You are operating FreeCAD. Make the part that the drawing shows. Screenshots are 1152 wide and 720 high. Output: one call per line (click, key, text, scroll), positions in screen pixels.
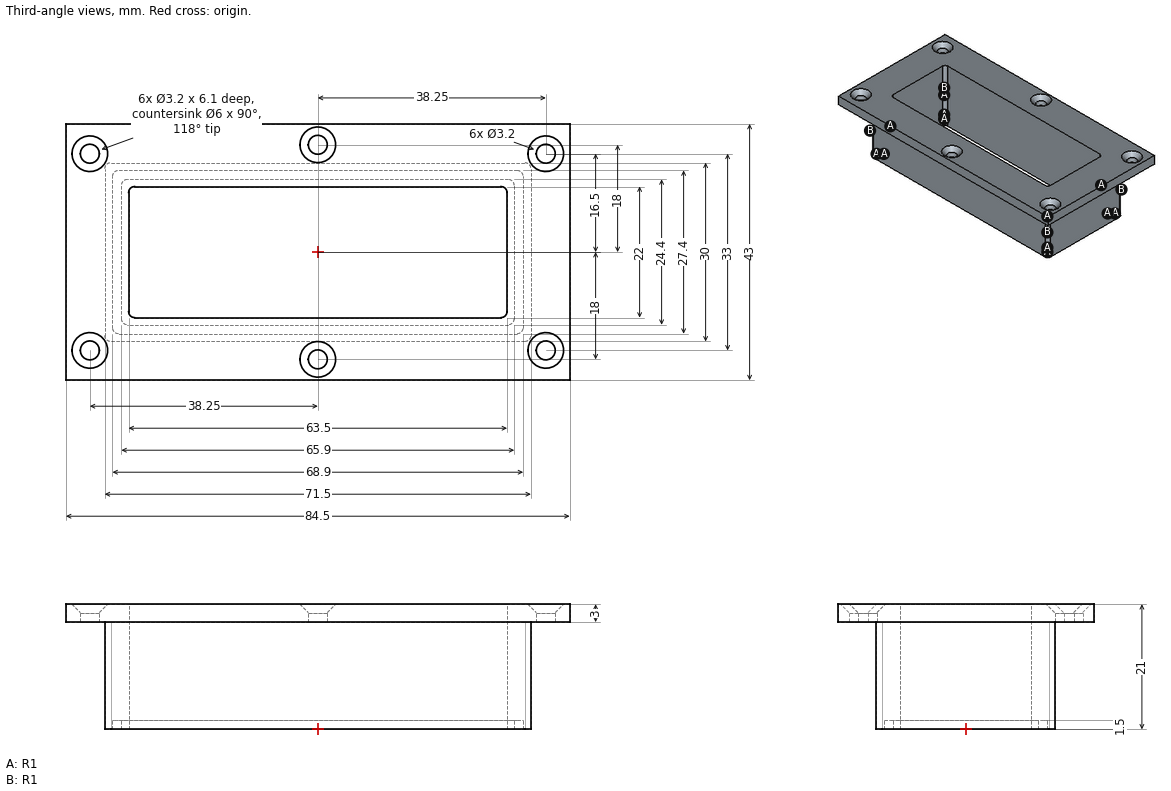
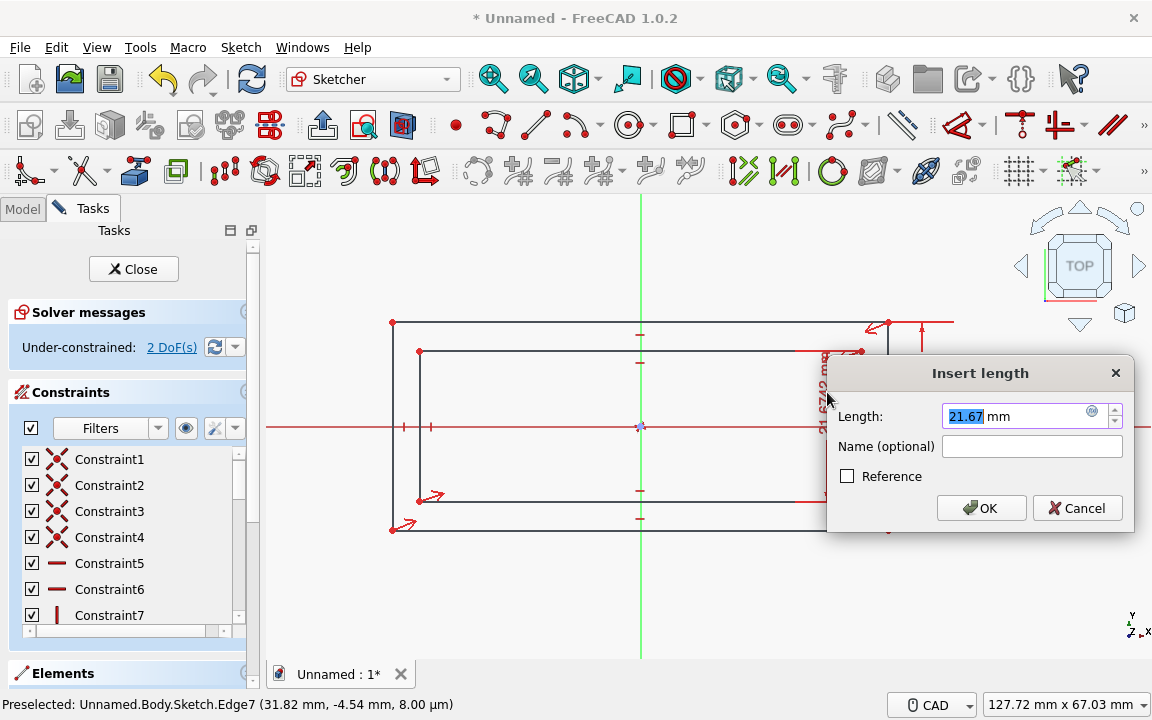
text(22)
key(Return)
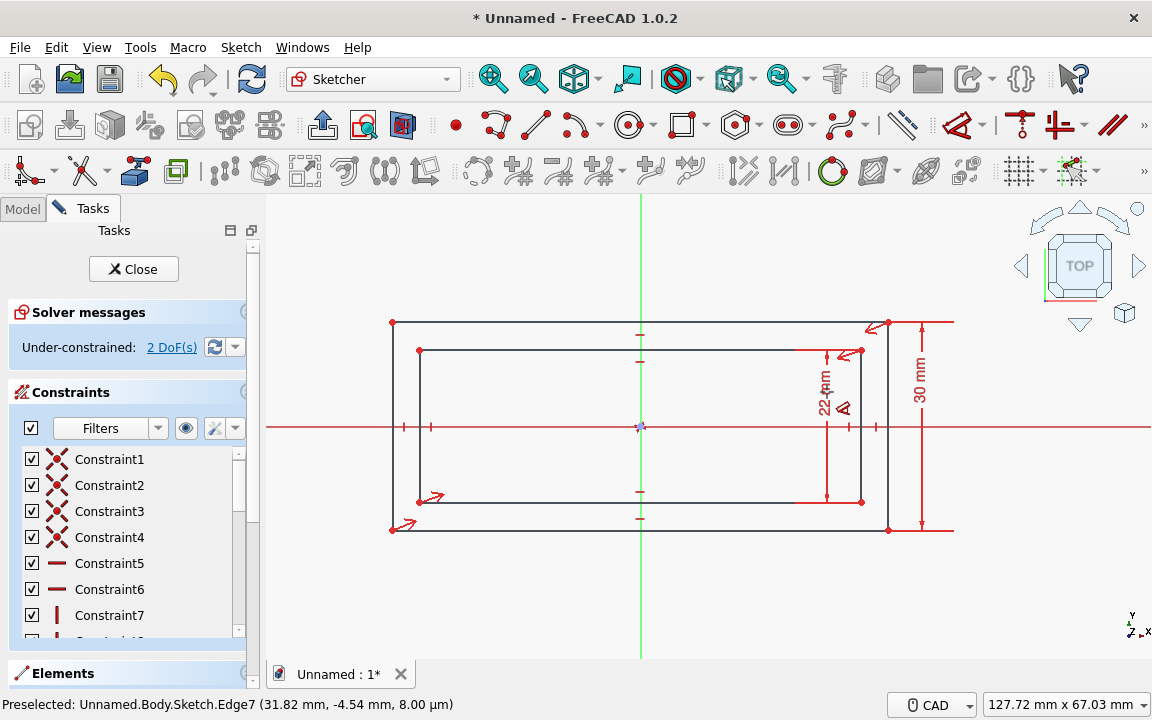
click(542, 531)
click(527, 565)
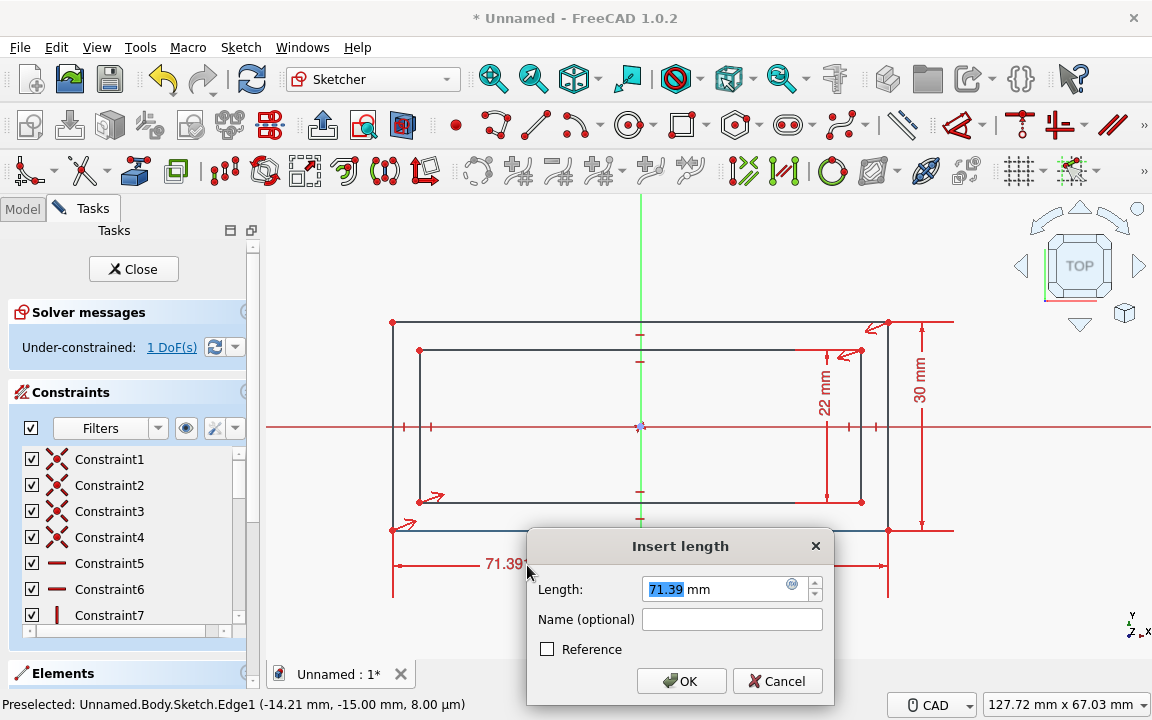
text(71.5)
key(Return)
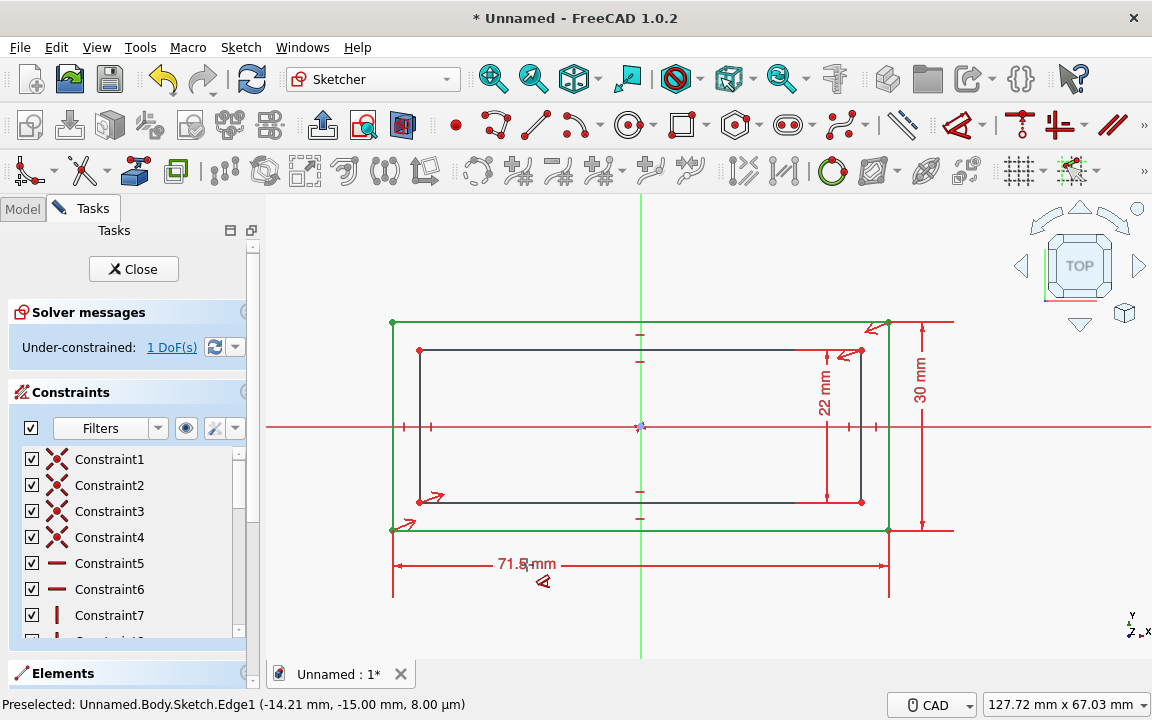
click(552, 503)
click(539, 469)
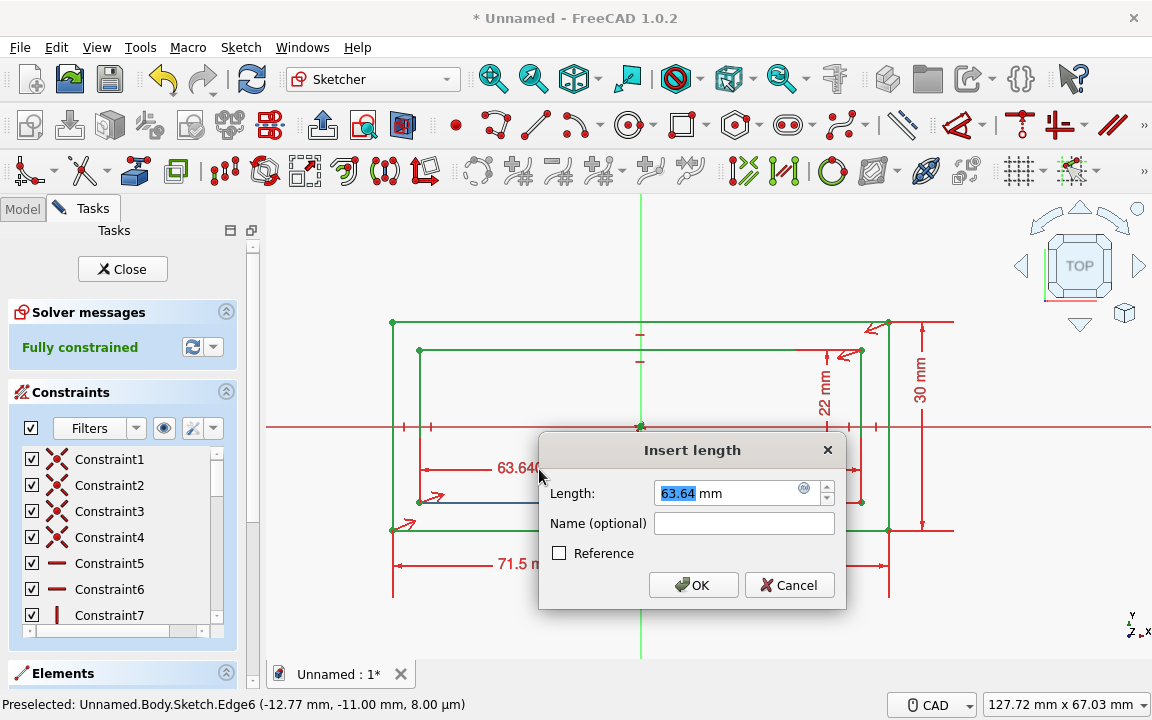
text(63.5)
key(Return)
key(Escape)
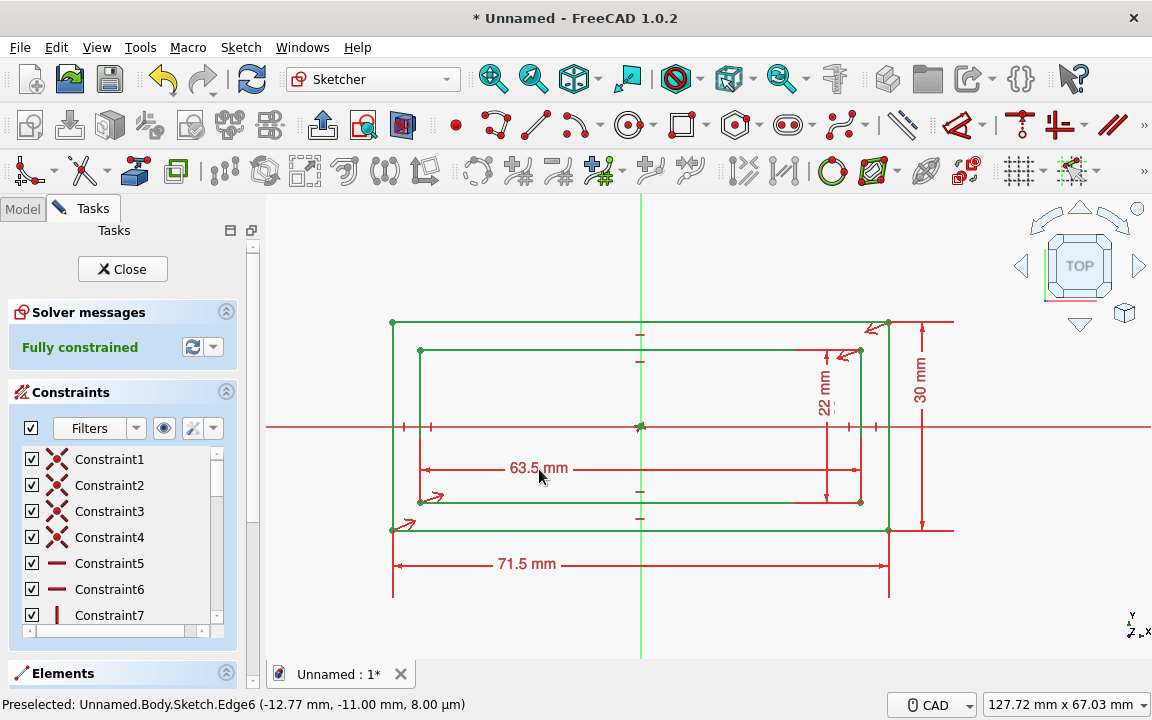
click(123, 269)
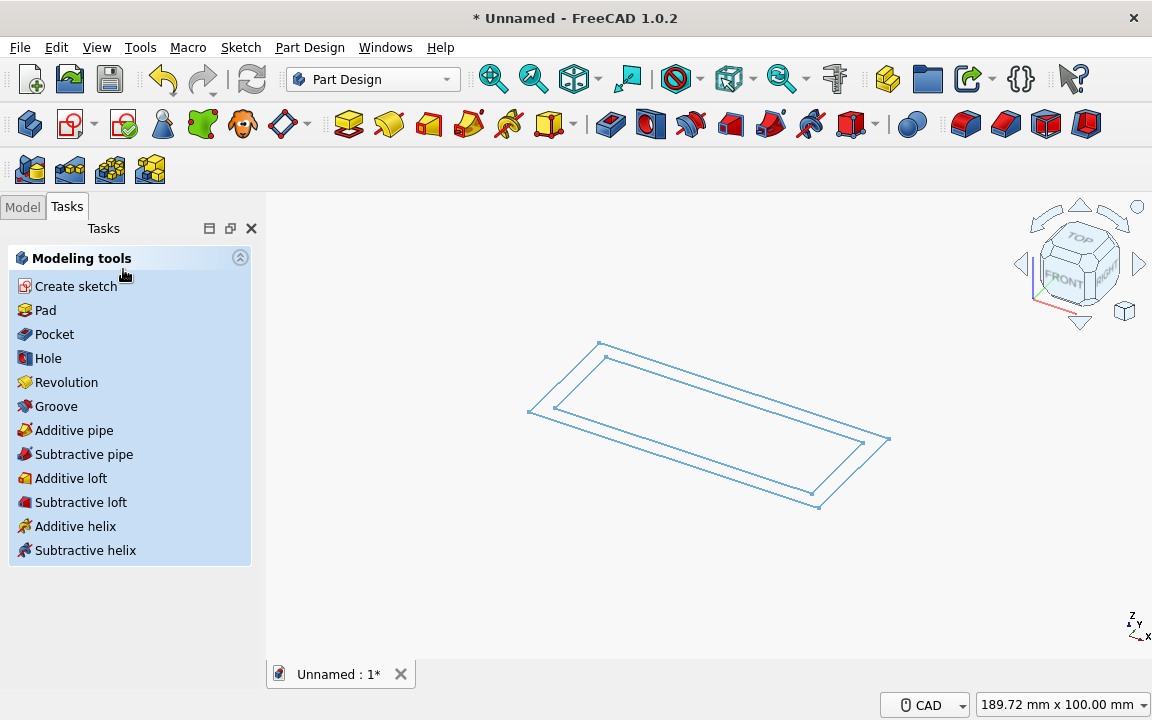
click(350, 124)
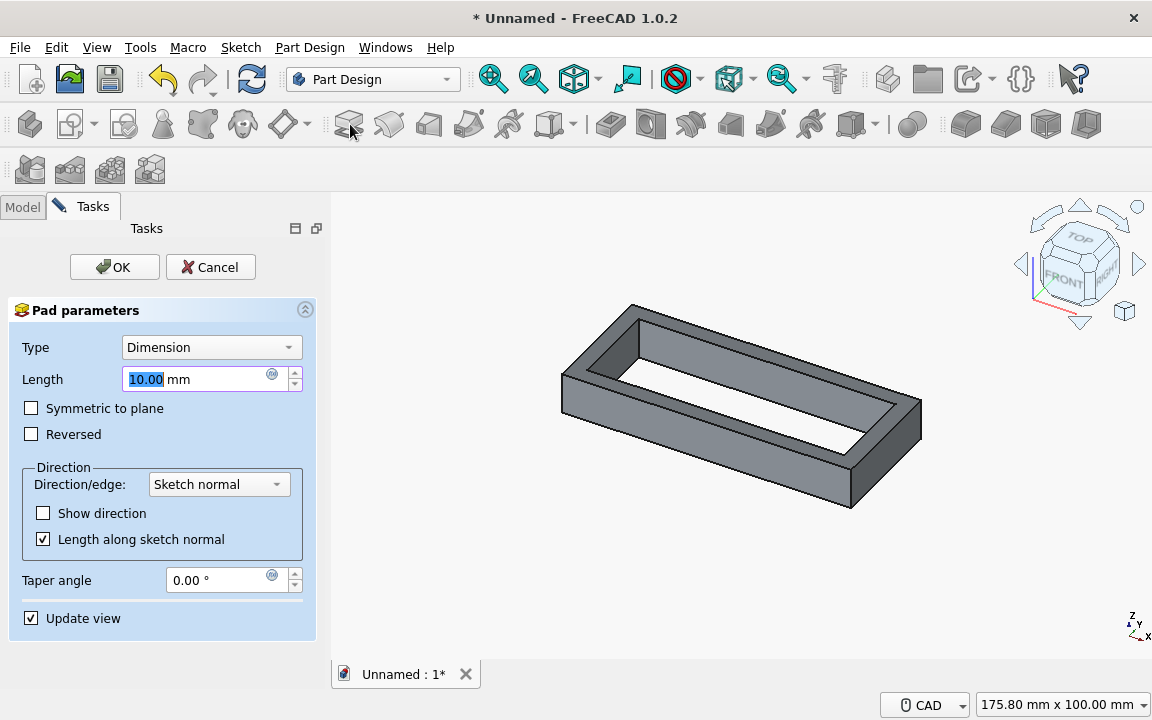
text(21)
key(Tab)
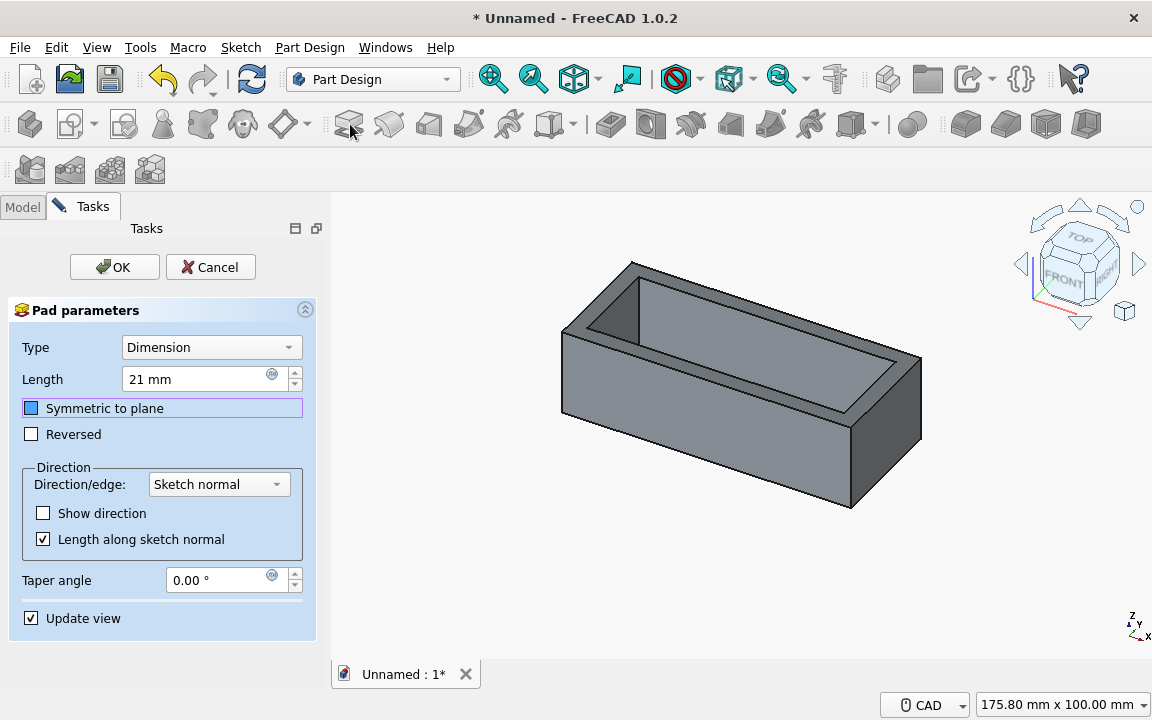
click(115, 267)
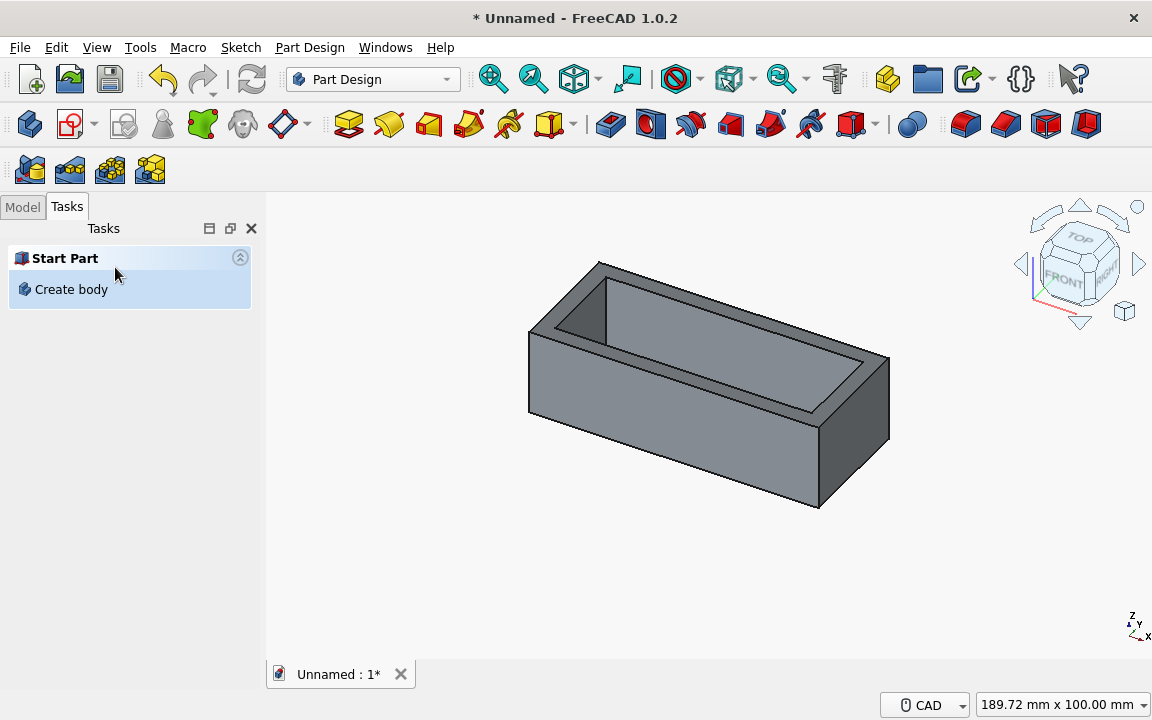
key(0)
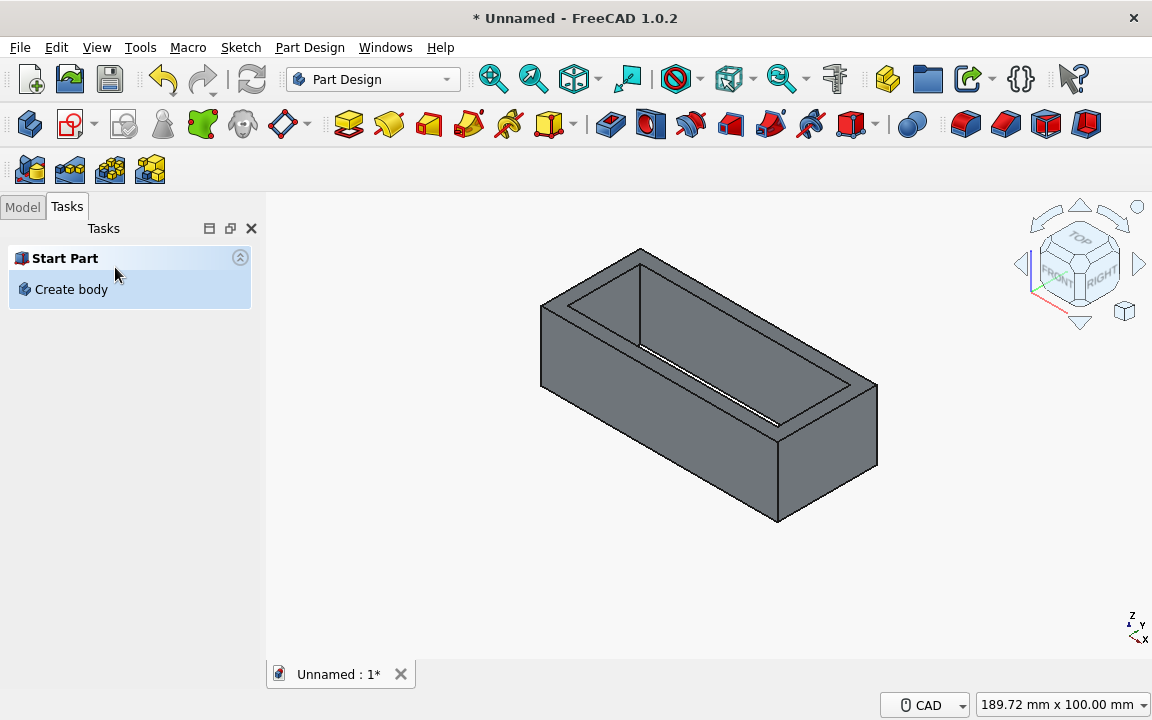
key(2)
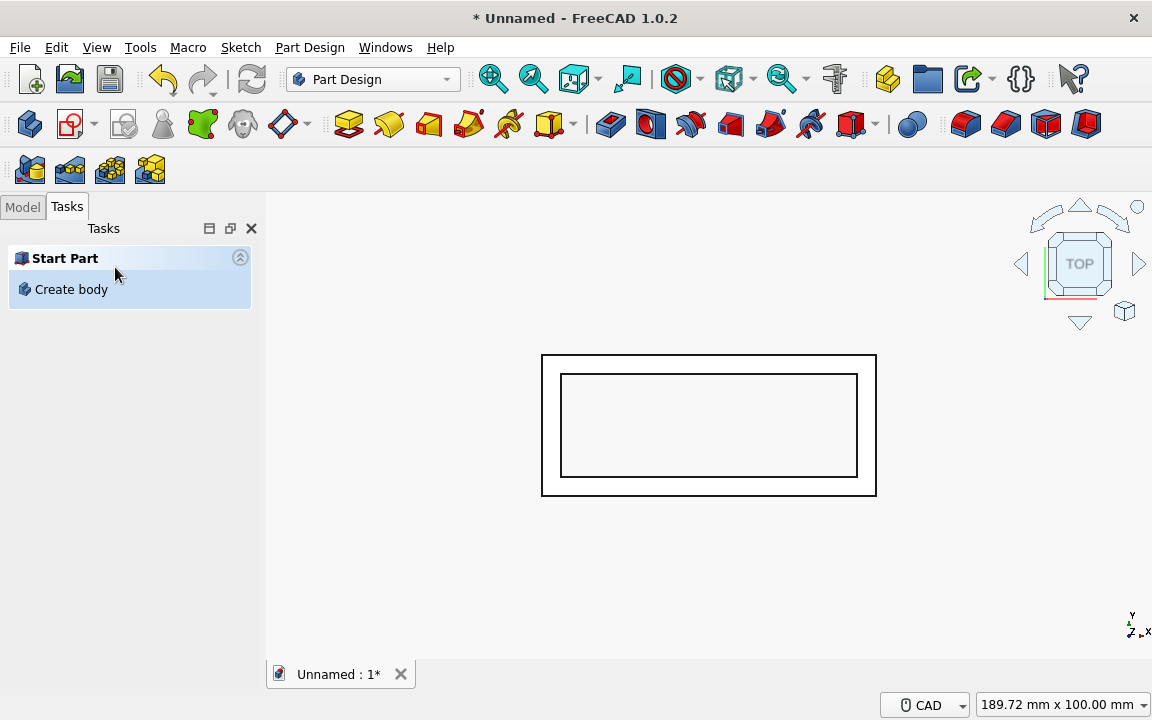
click(494, 80)